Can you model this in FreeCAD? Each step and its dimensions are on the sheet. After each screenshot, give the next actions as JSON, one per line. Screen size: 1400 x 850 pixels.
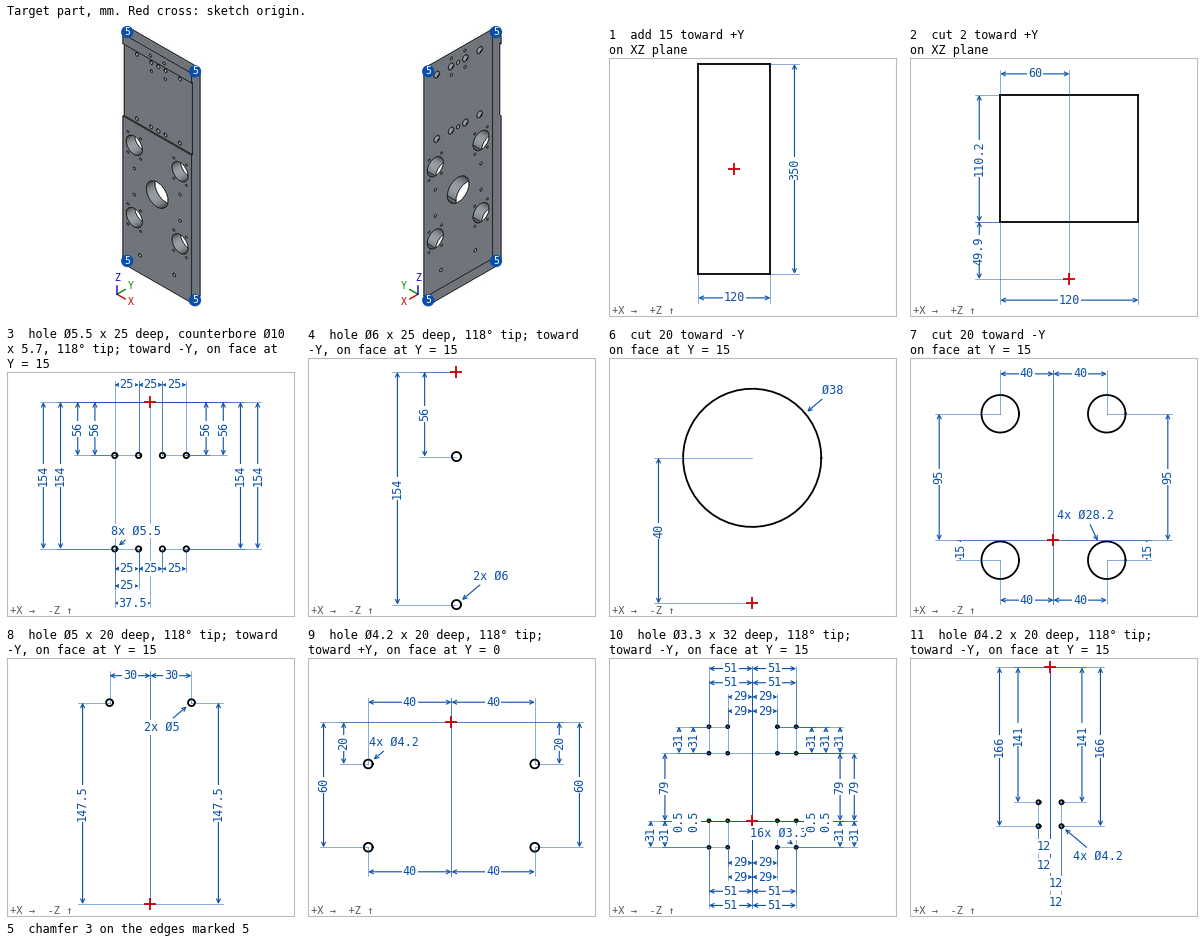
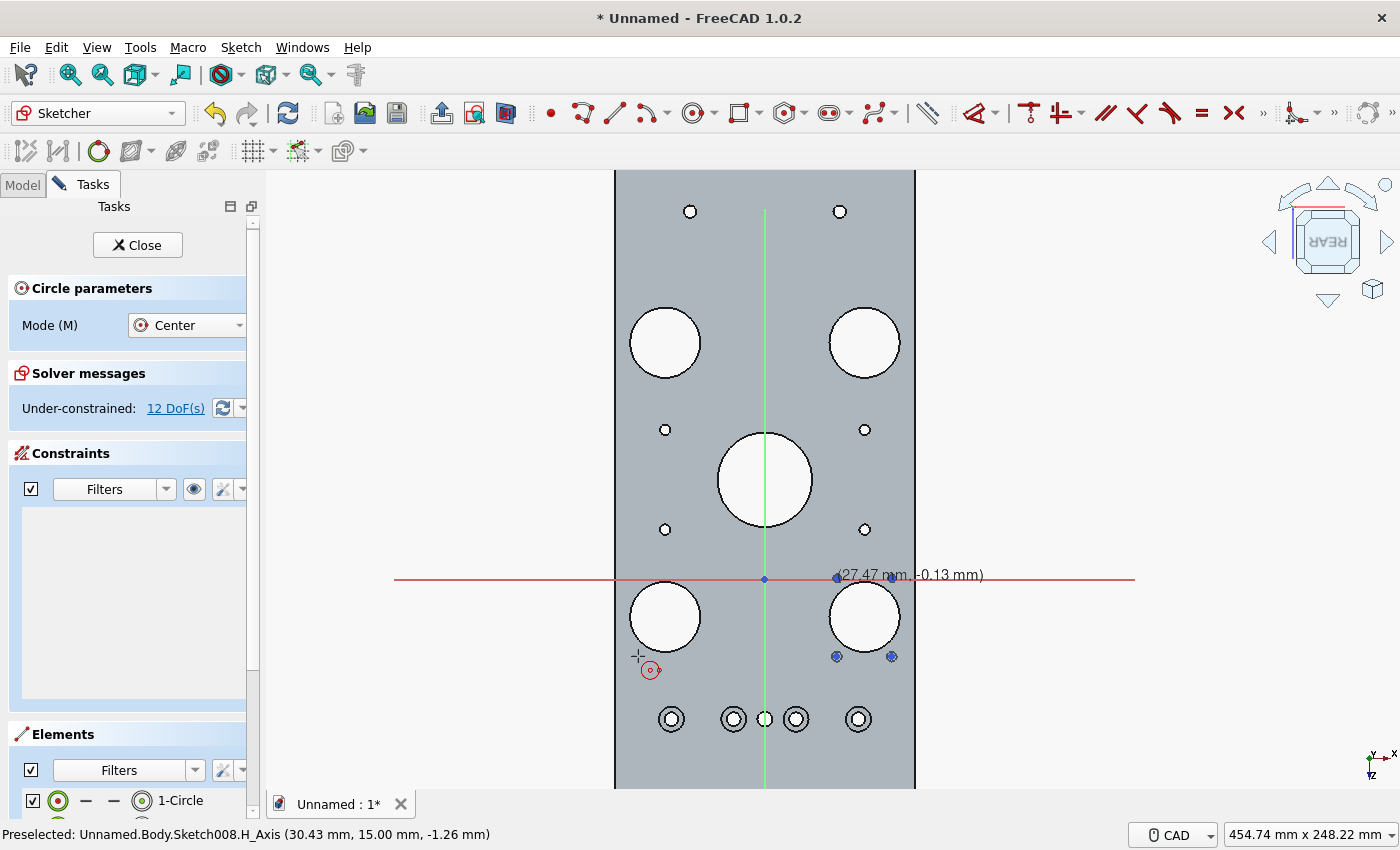
{"action": "left_click", "coordinate": [638, 656]}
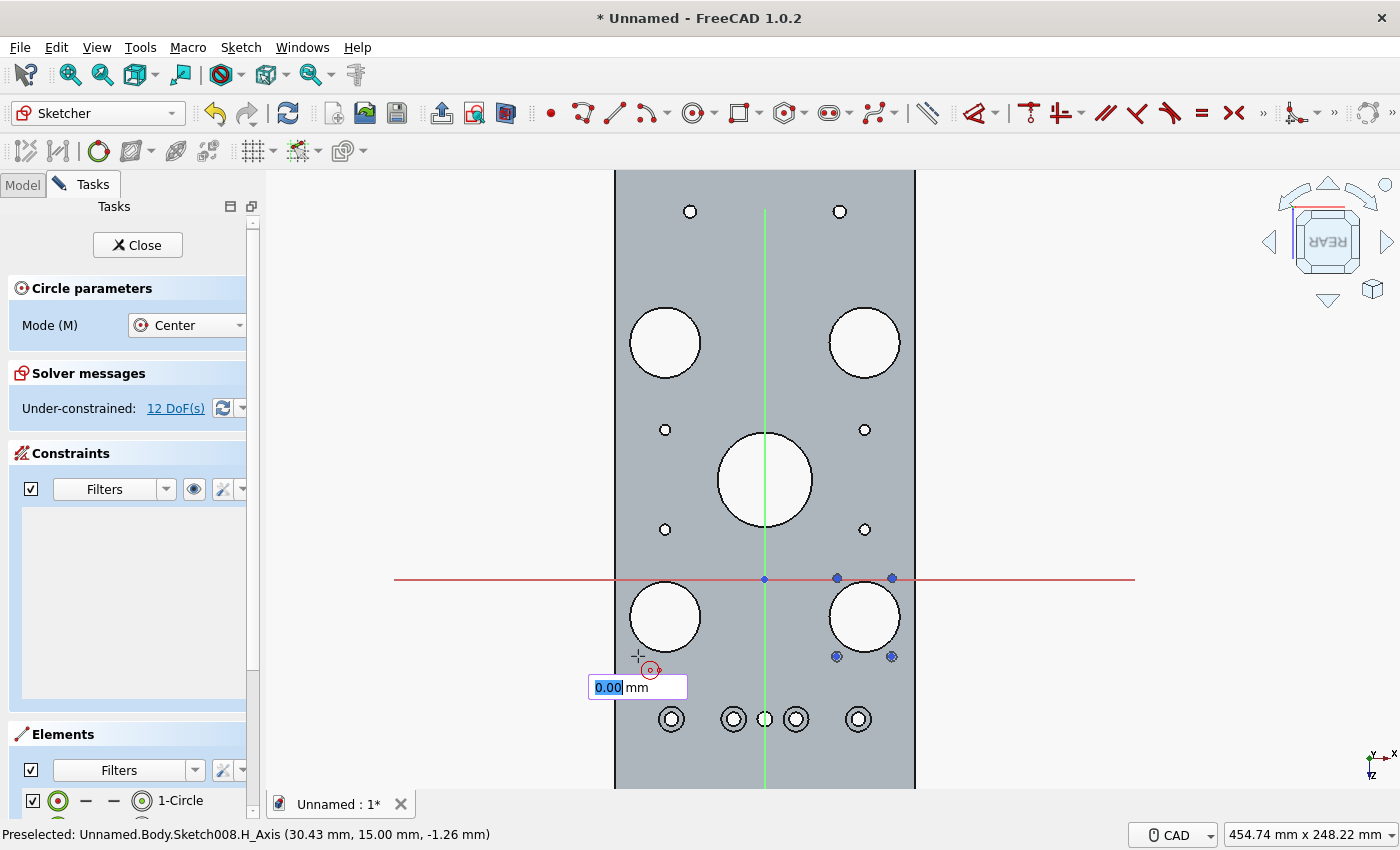
{"action": "scroll", "coordinate": [641, 653], "scroll_direction": "up", "scroll_amount": 7}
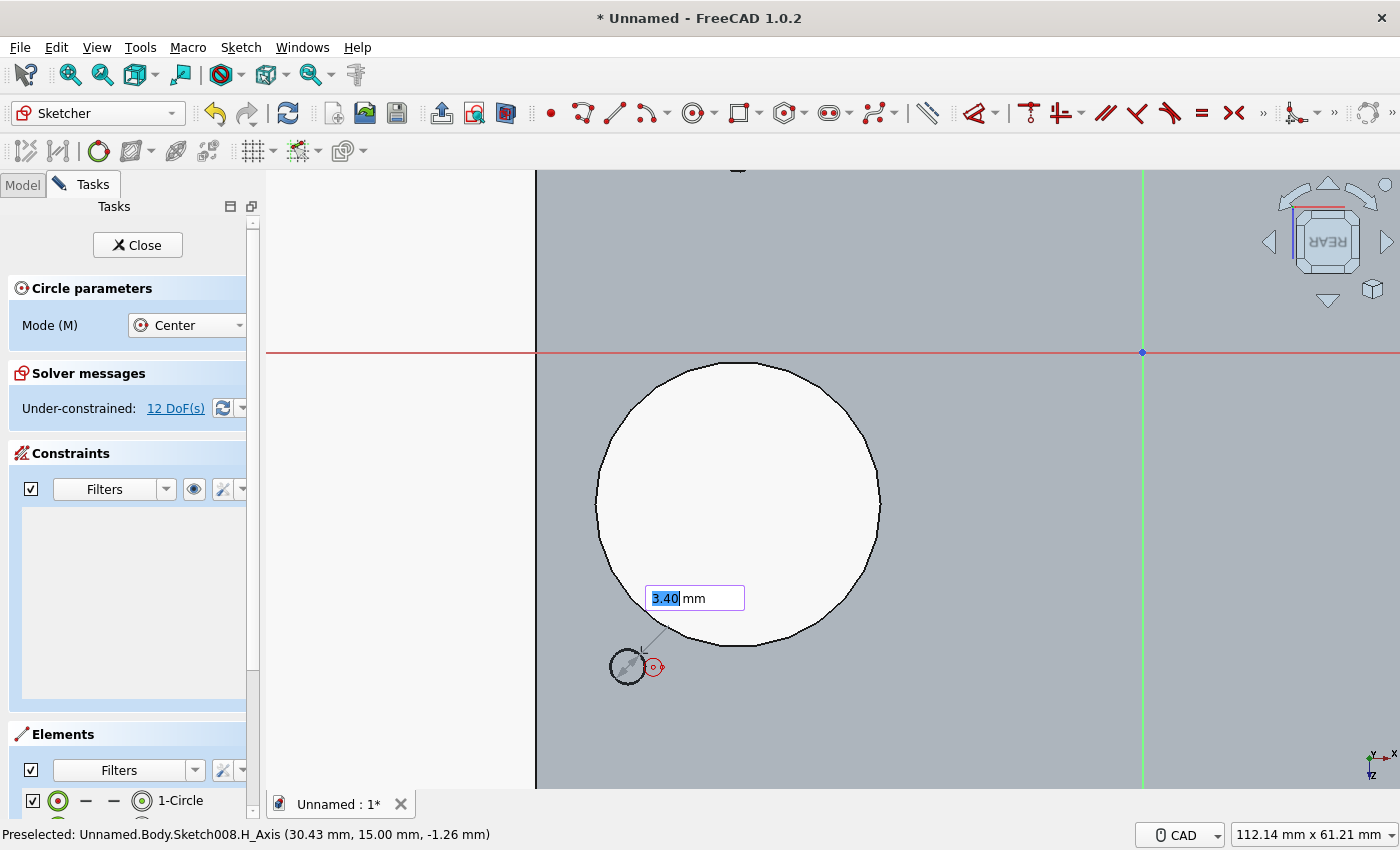
{"action": "left_click", "coordinate": [639, 649]}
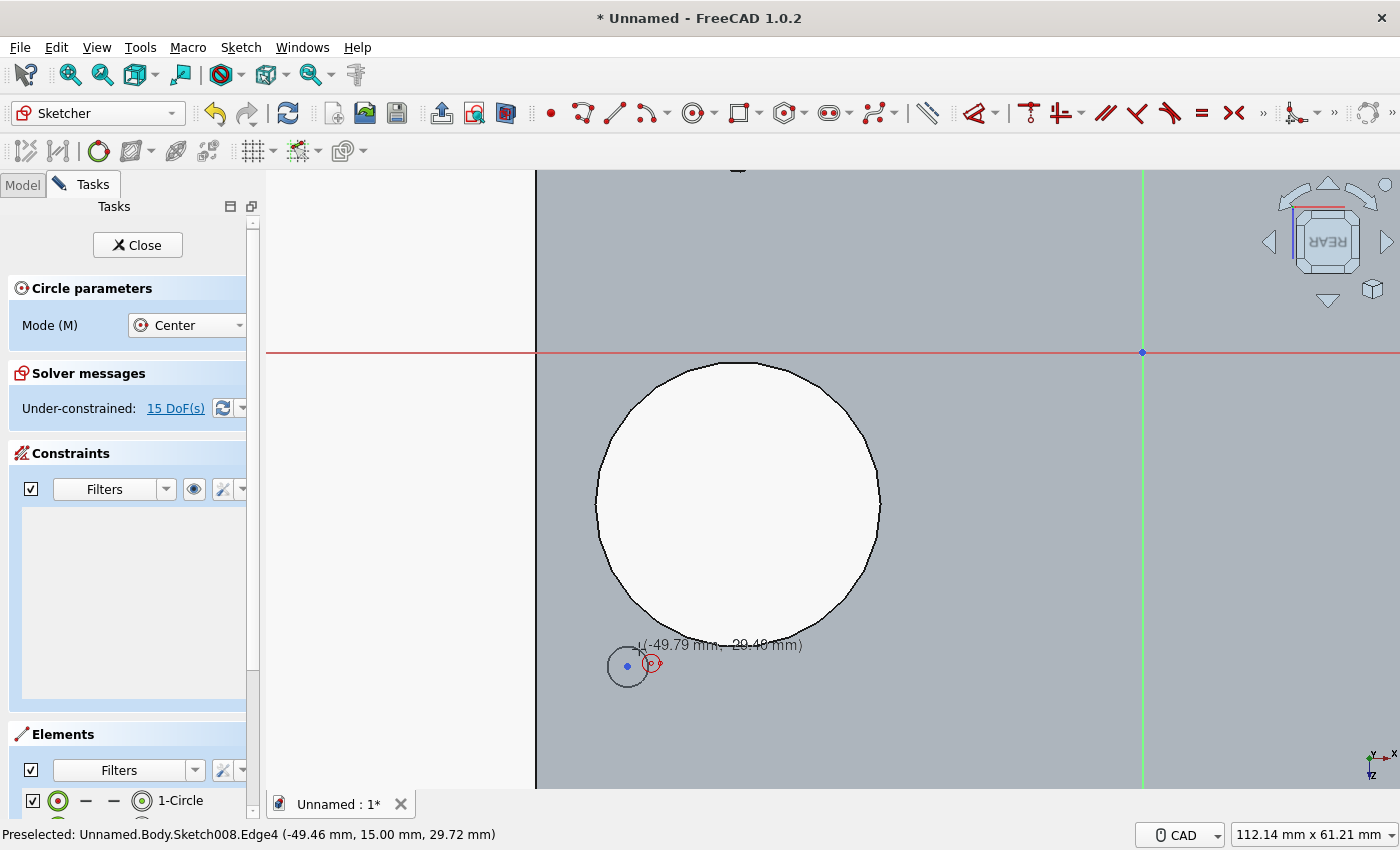
{"action": "scroll", "coordinate": [849, 661], "scroll_direction": "up", "scroll_amount": 2}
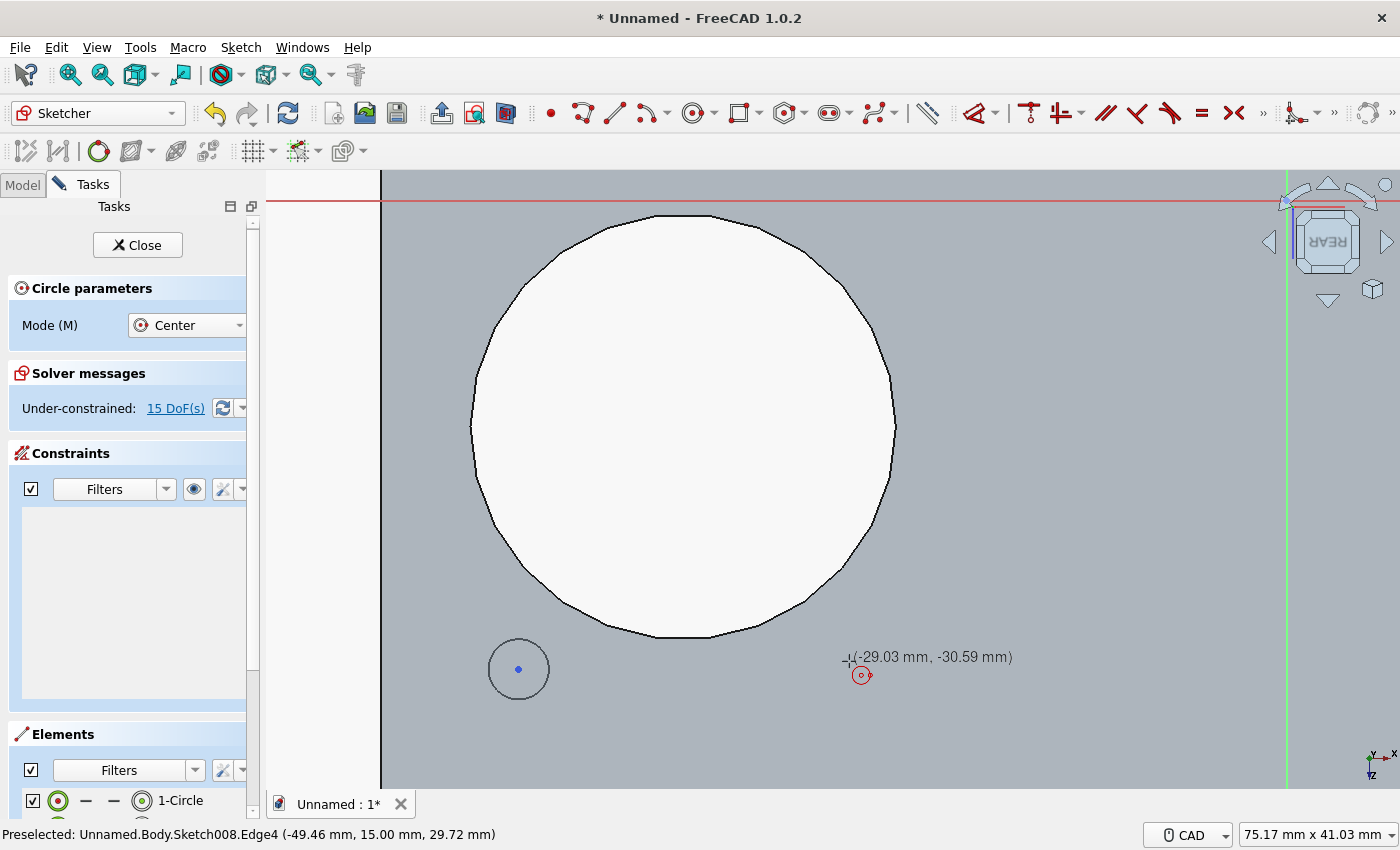
{"action": "scroll", "coordinate": [661, 654], "scroll_direction": "down", "scroll_amount": 9}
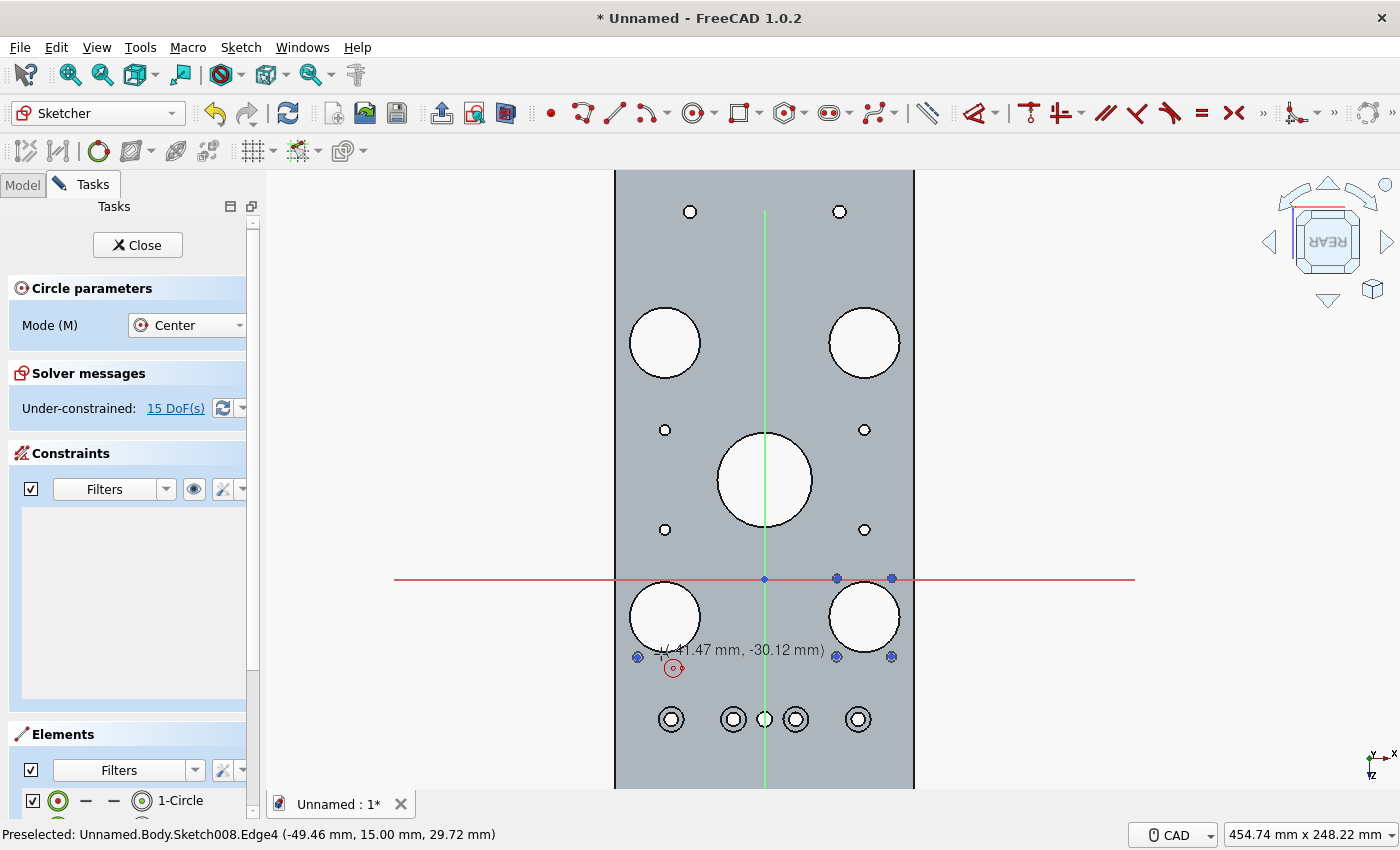
{"action": "left_click", "coordinate": [692, 656]}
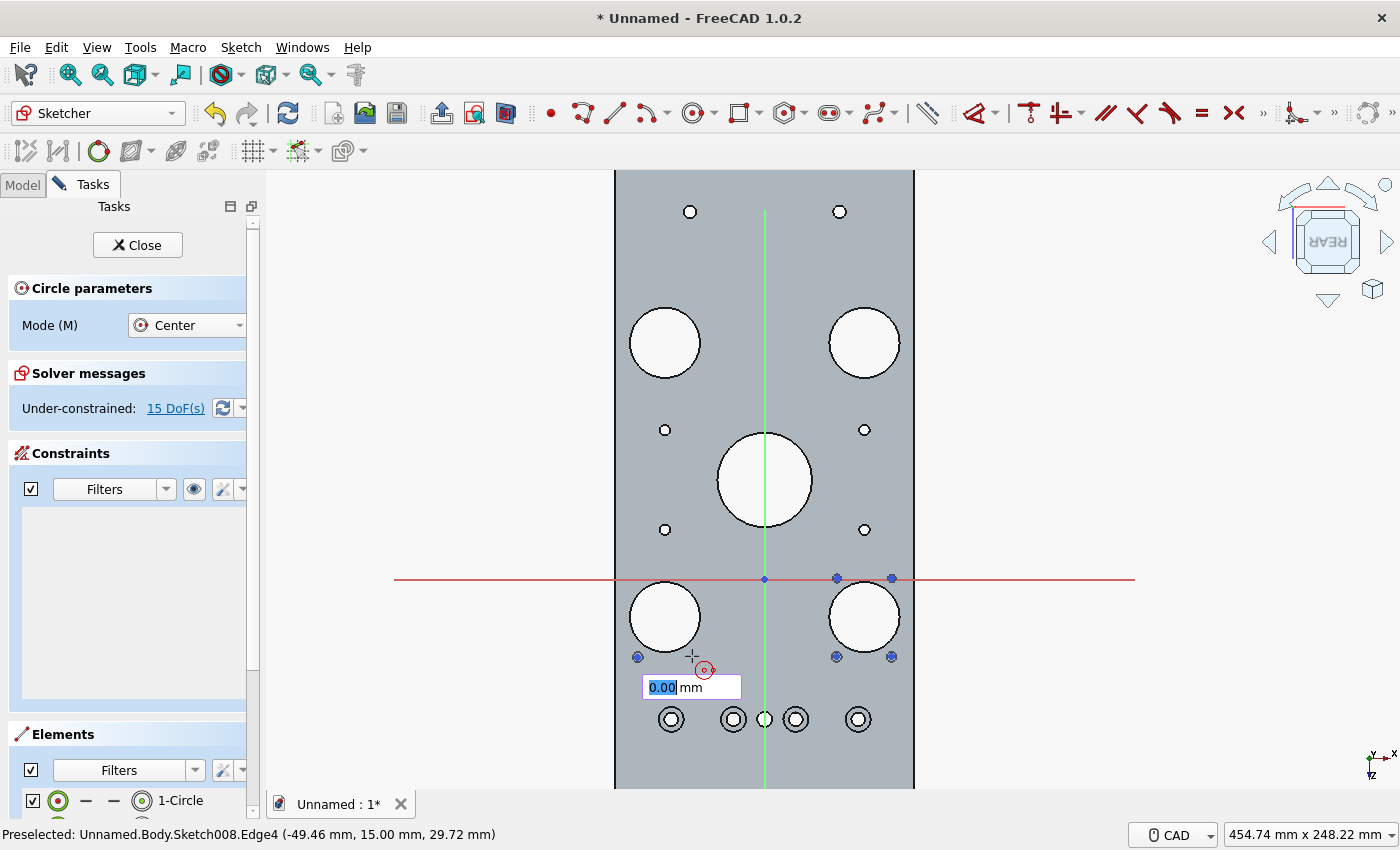
{"action": "scroll", "coordinate": [695, 653], "scroll_direction": "up", "scroll_amount": 7}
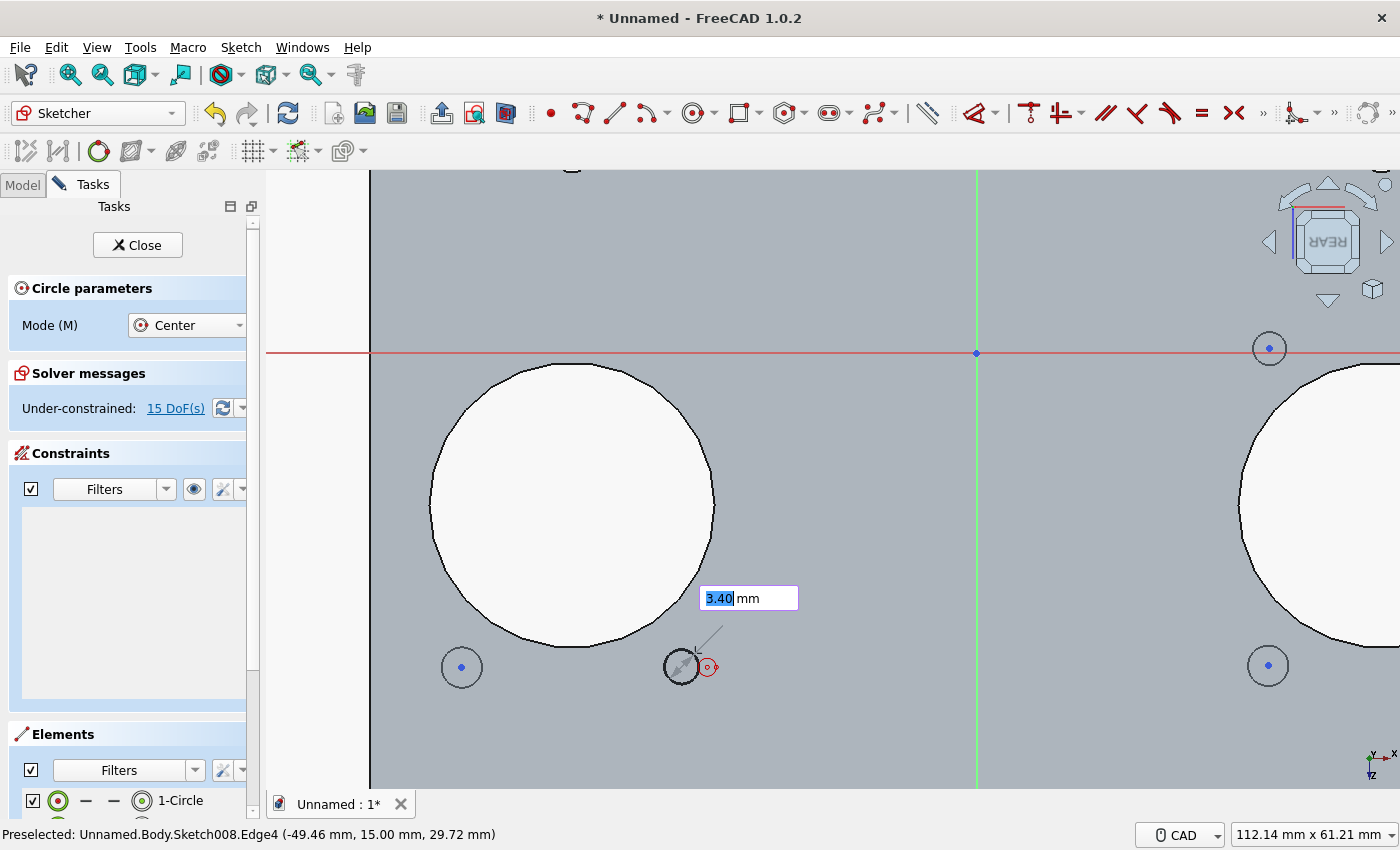
{"action": "left_click", "coordinate": [695, 650]}